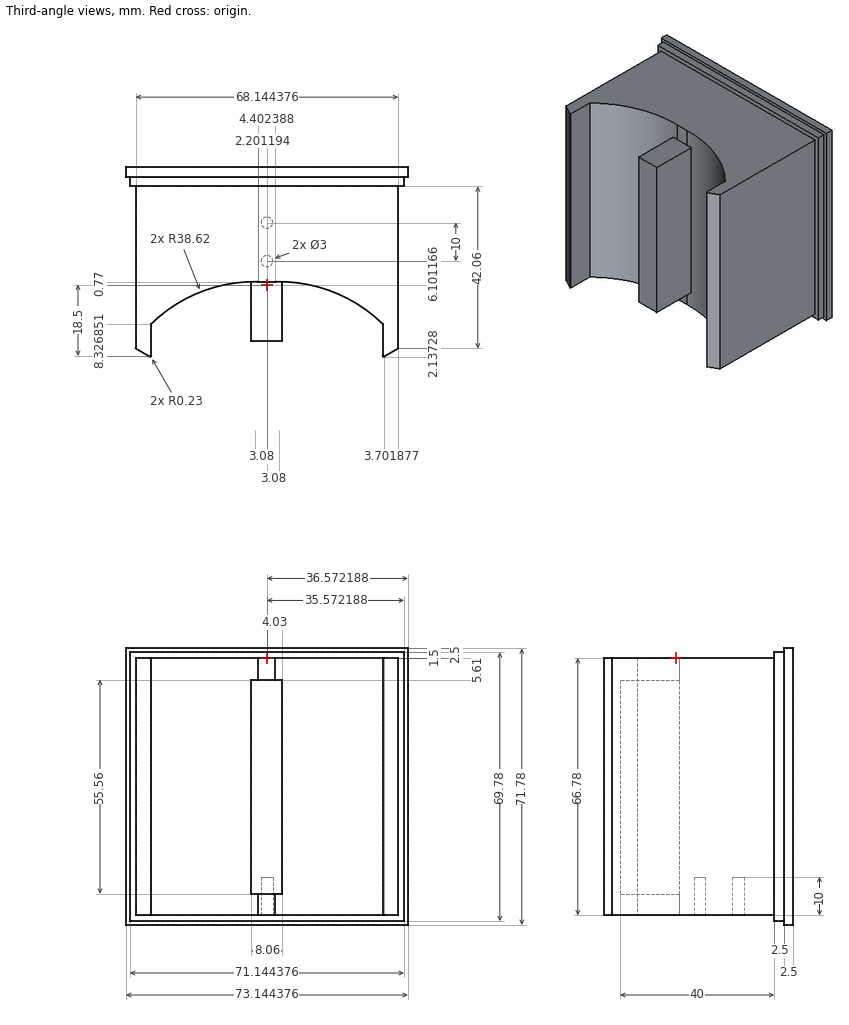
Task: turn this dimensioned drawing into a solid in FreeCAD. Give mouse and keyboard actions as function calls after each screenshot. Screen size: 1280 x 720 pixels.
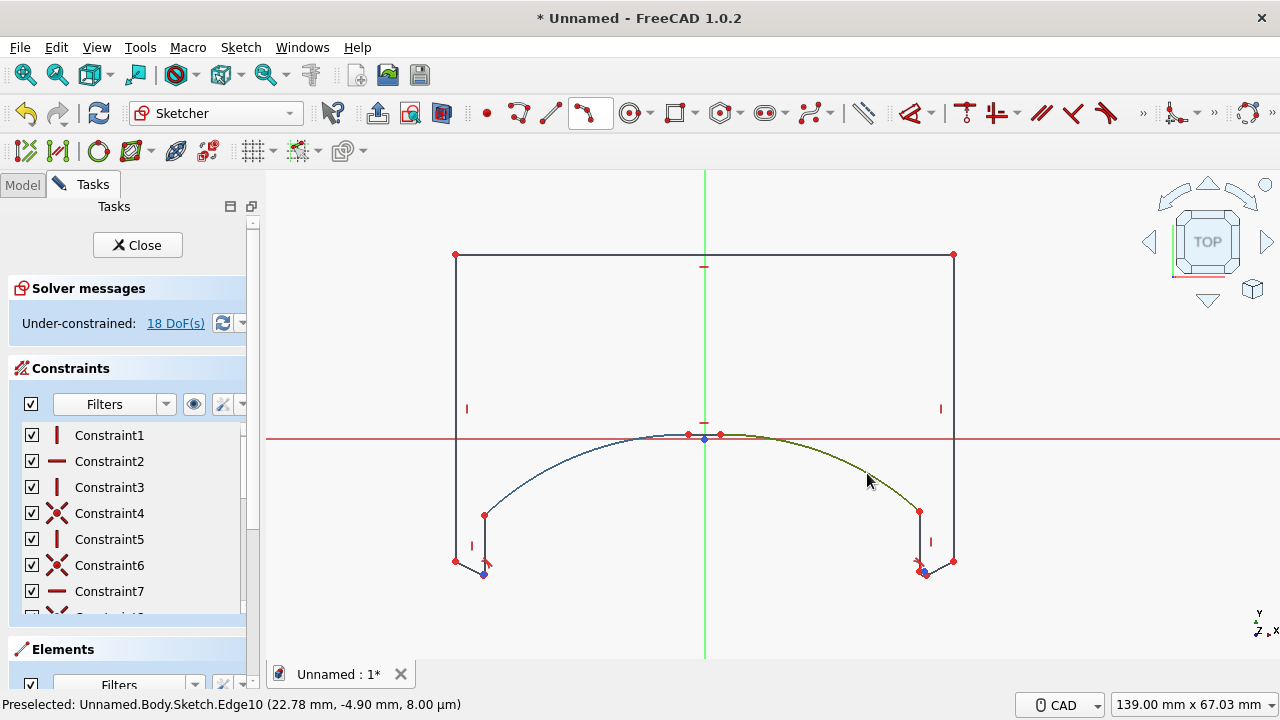
key(e)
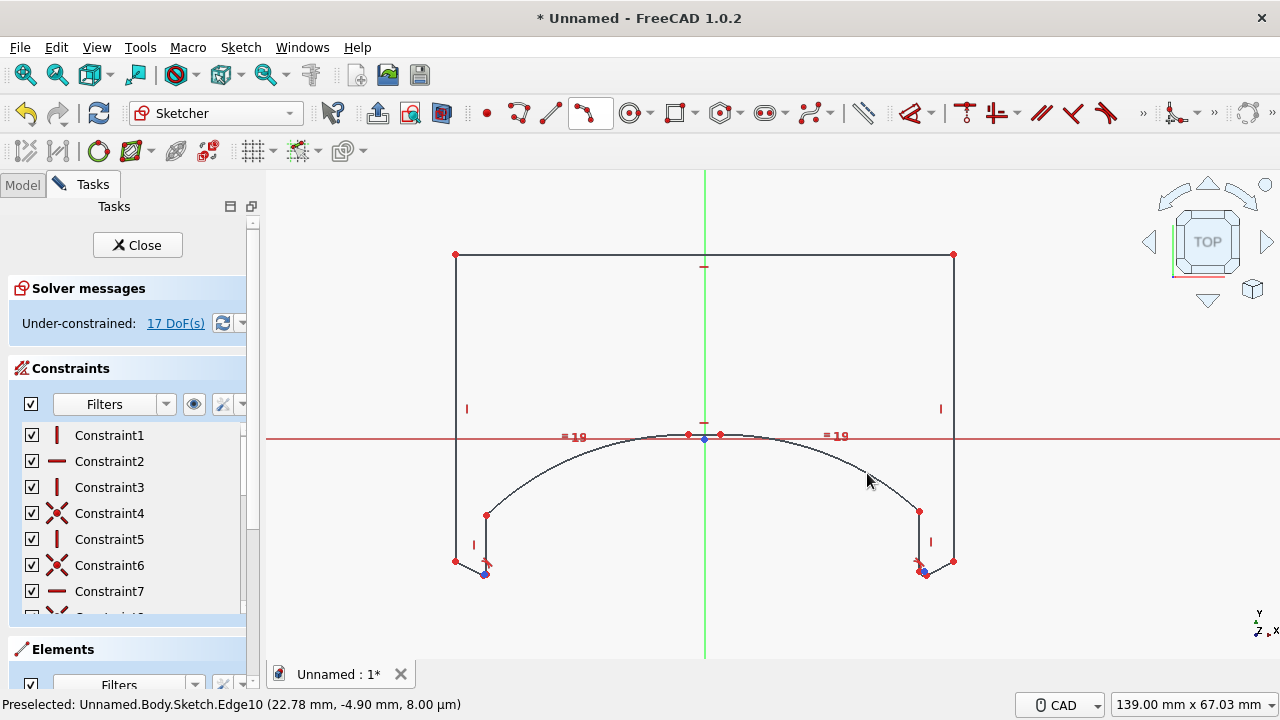
scroll(922, 575, up, 6)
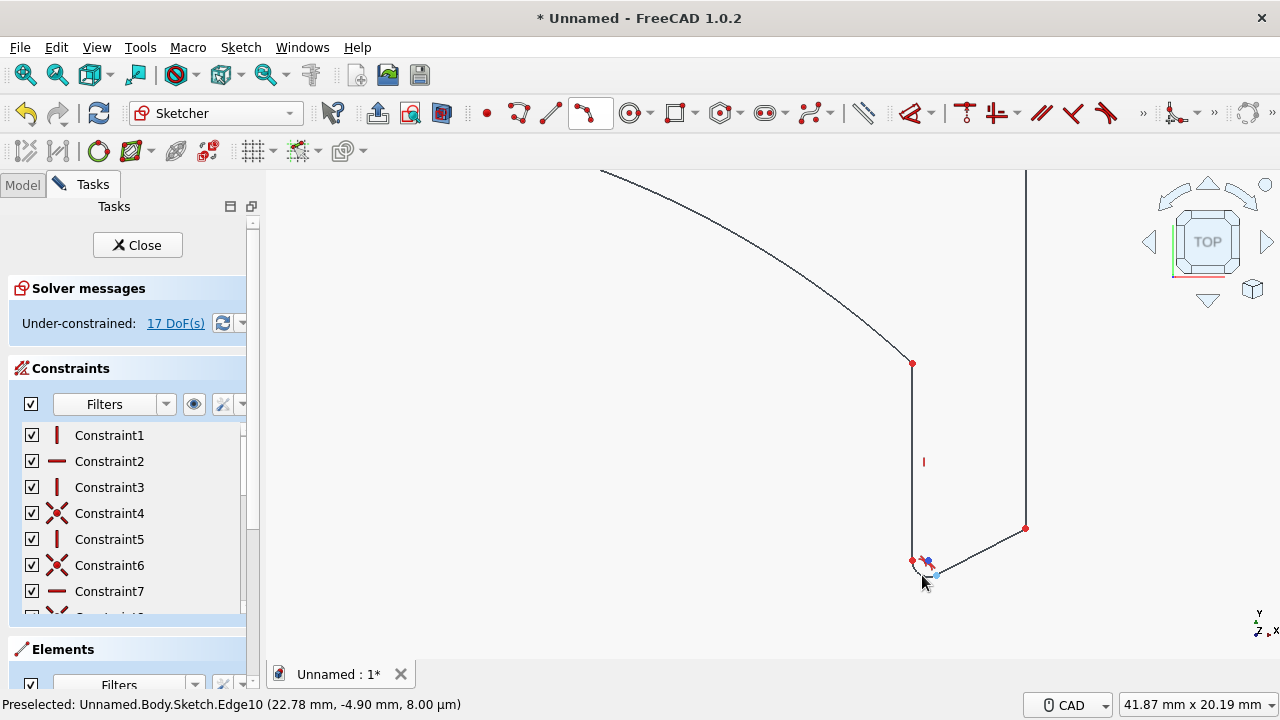
click(920, 575)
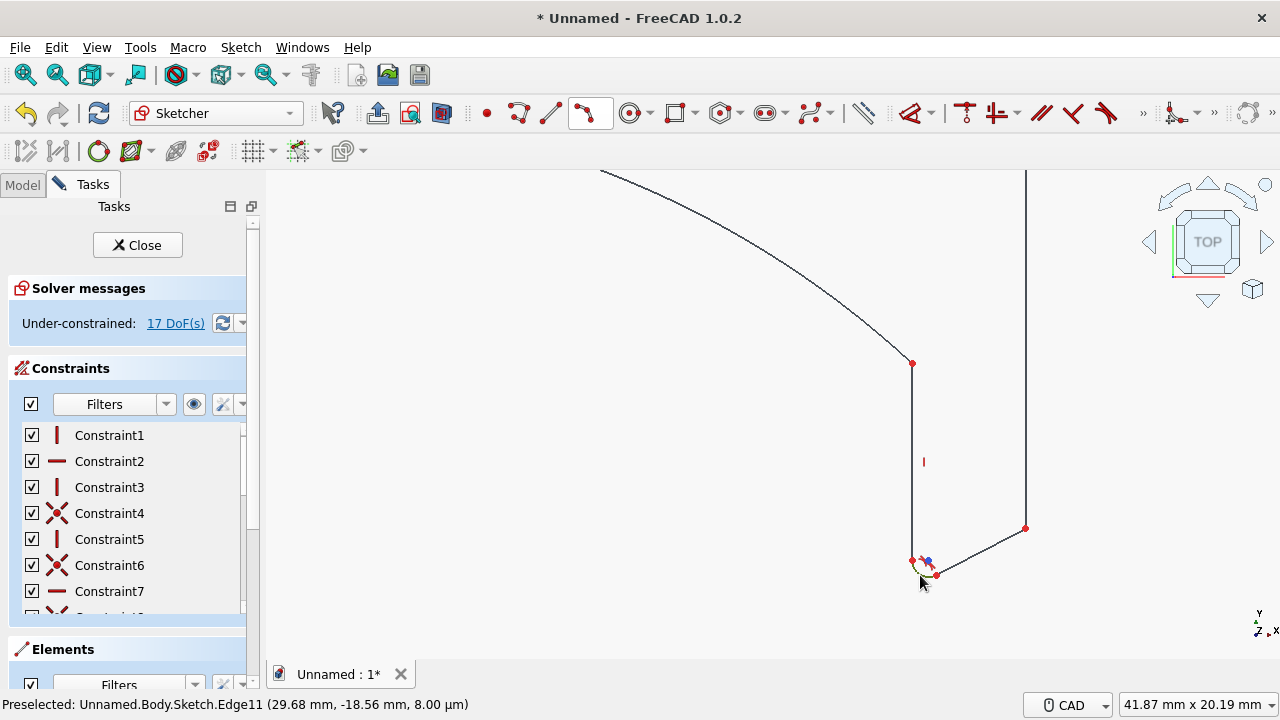
scroll(923, 576, down, 6)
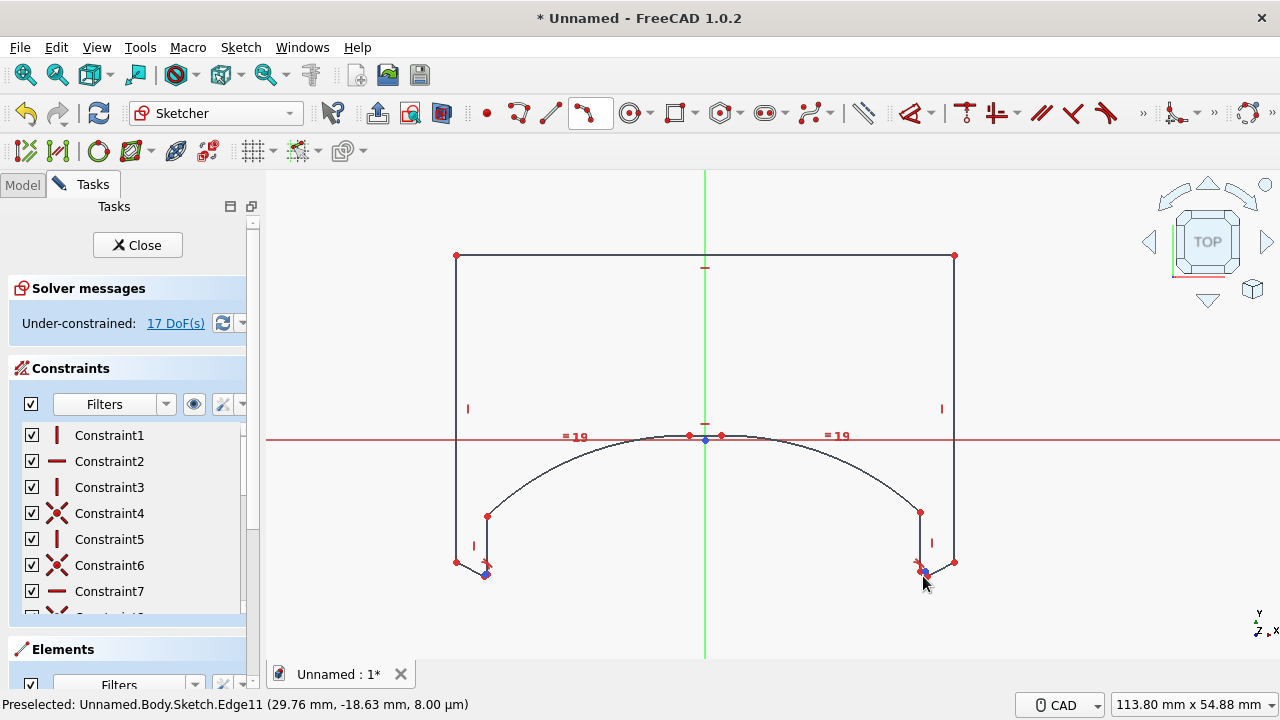
scroll(486, 576, up, 10)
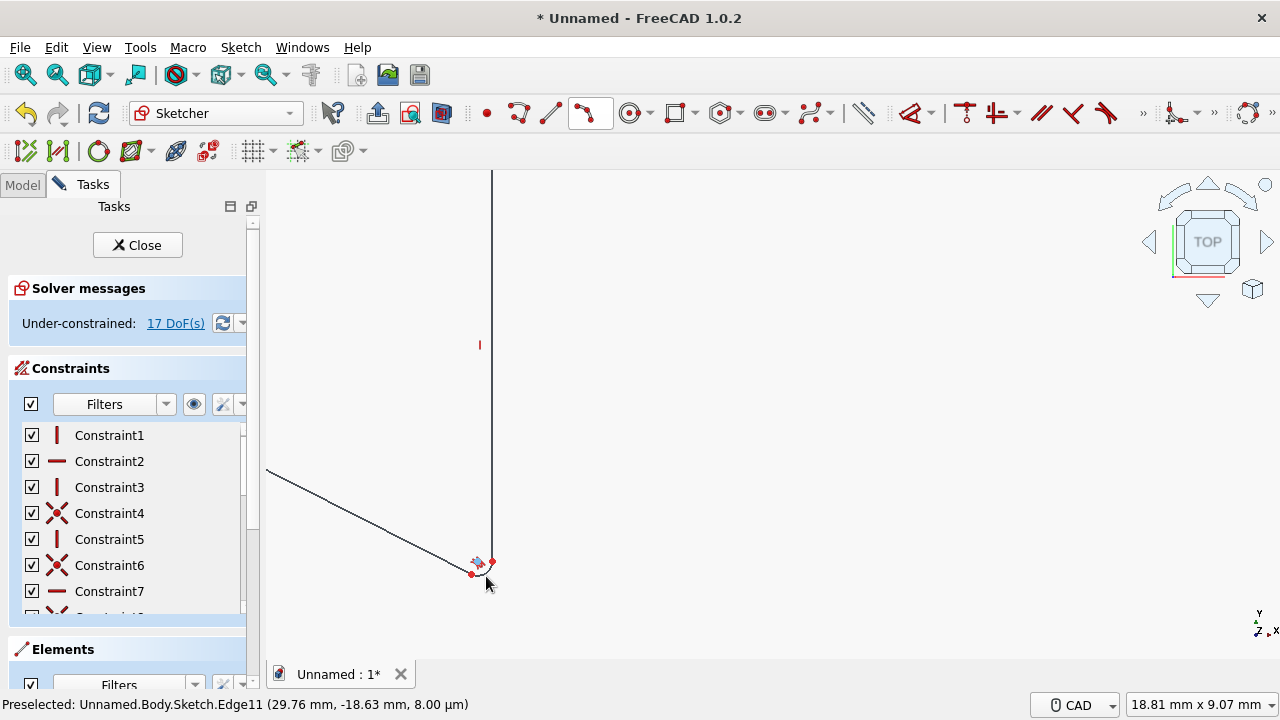
click(485, 574)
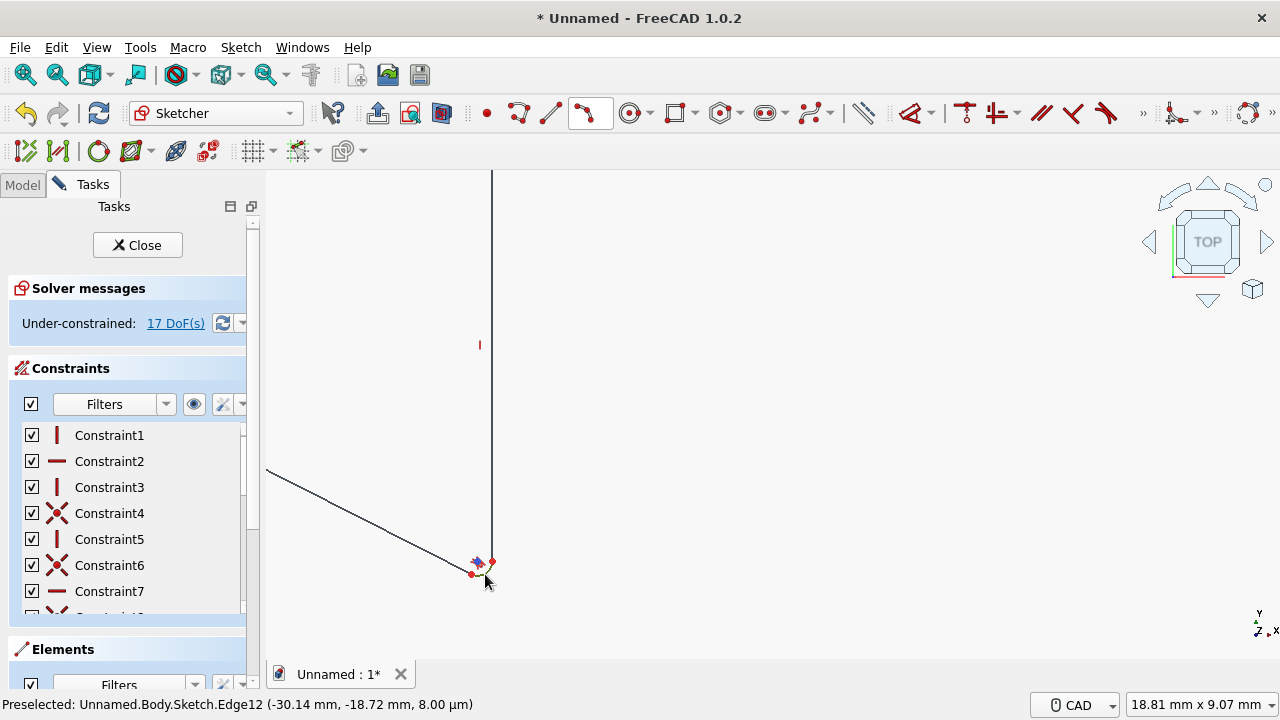
key(e)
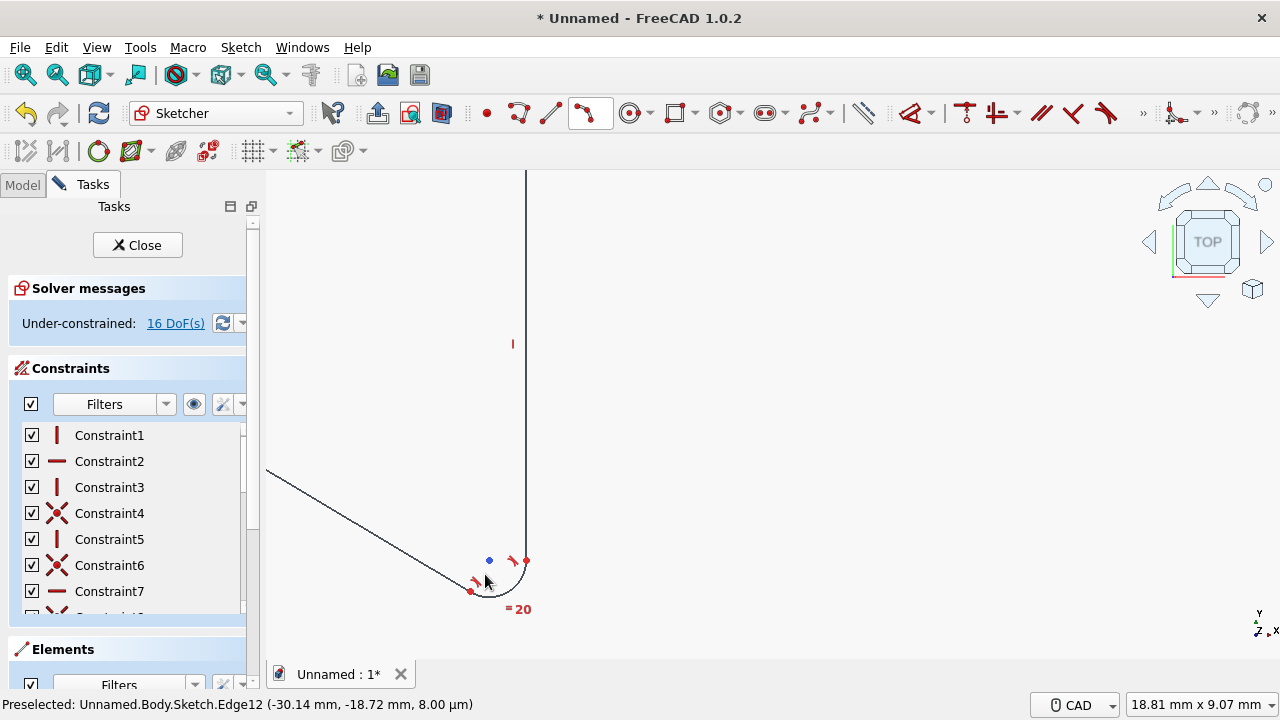
click(910, 114)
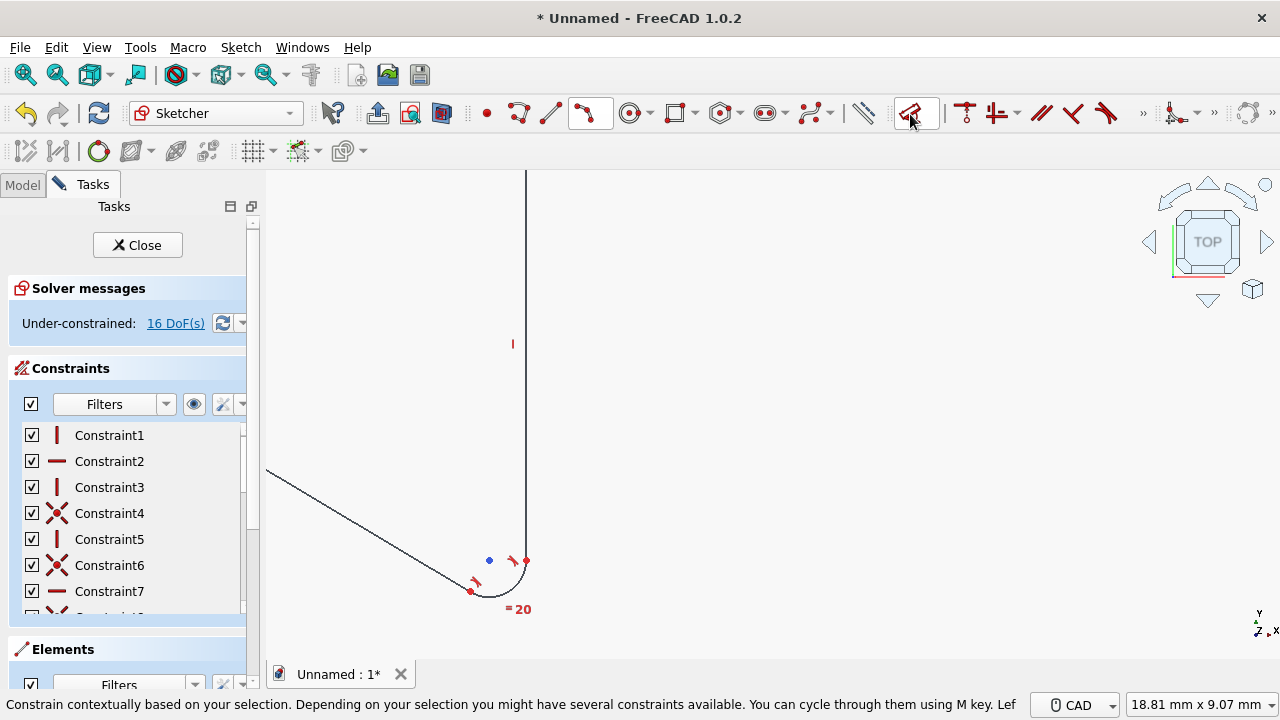
scroll(485, 576, down, 10)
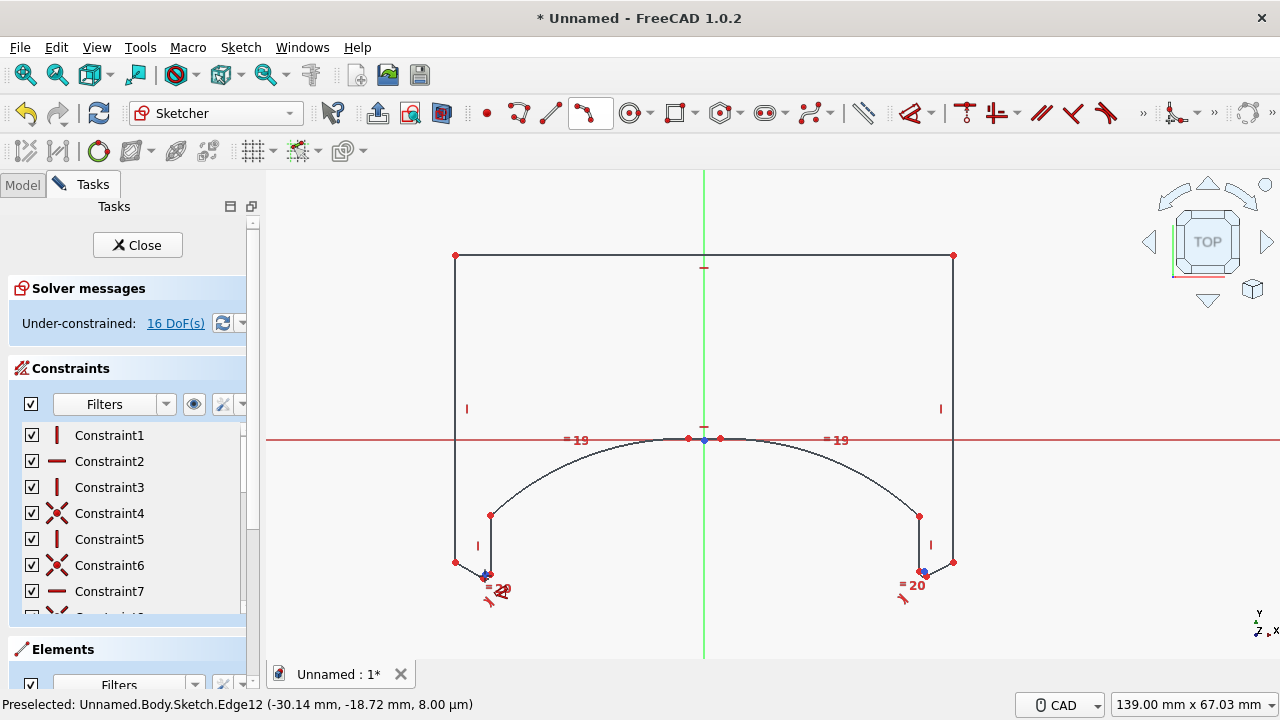
scroll(624, 445, up, 5)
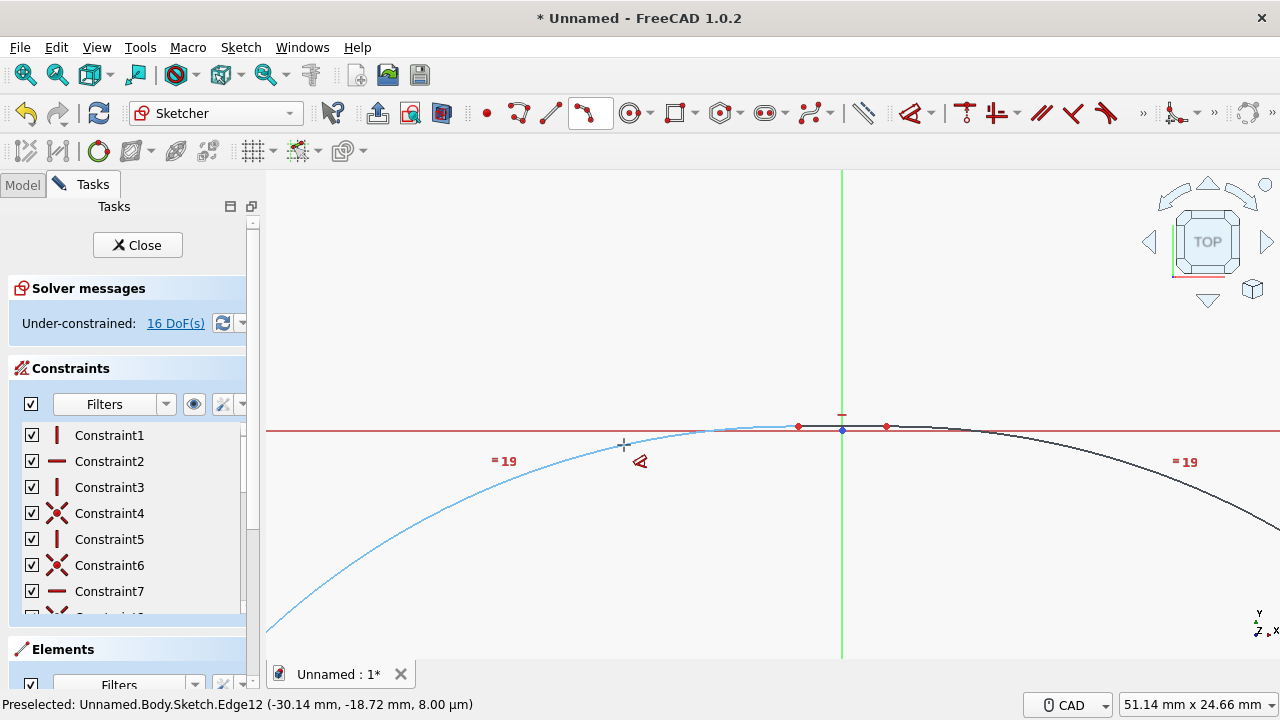
click(622, 445)
click(615, 414)